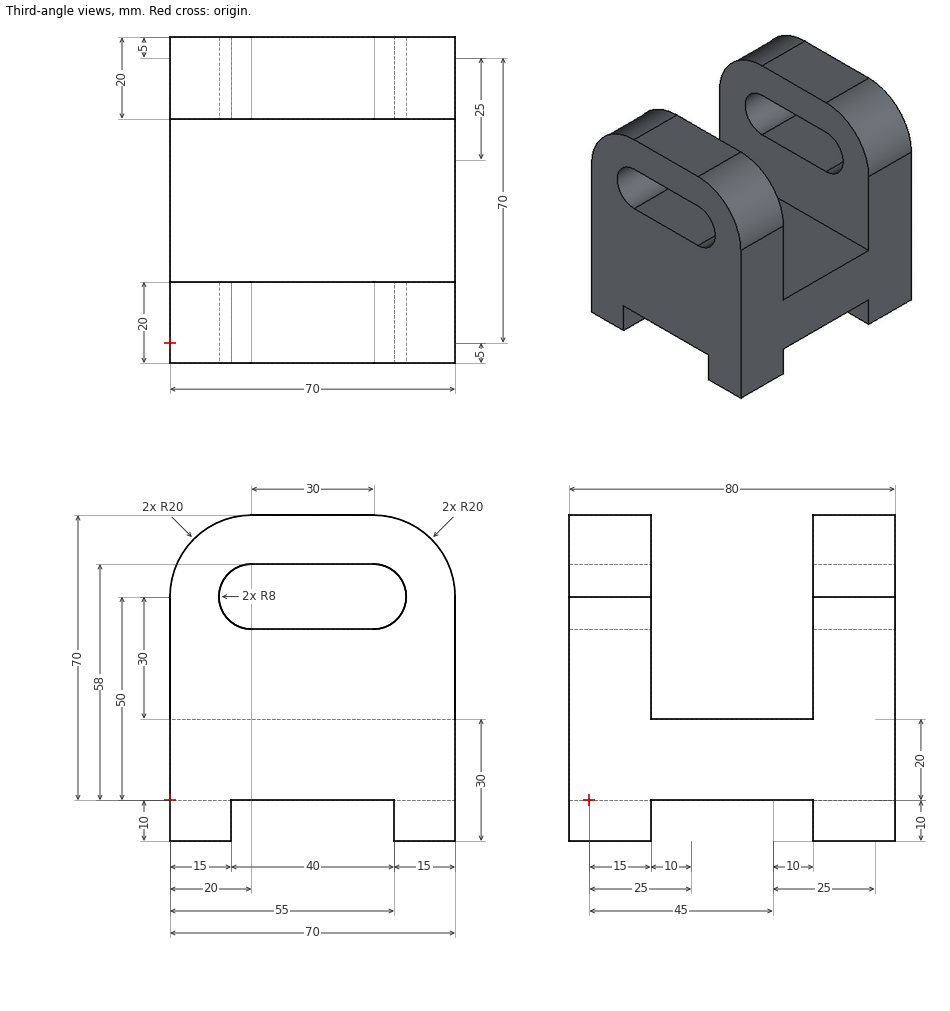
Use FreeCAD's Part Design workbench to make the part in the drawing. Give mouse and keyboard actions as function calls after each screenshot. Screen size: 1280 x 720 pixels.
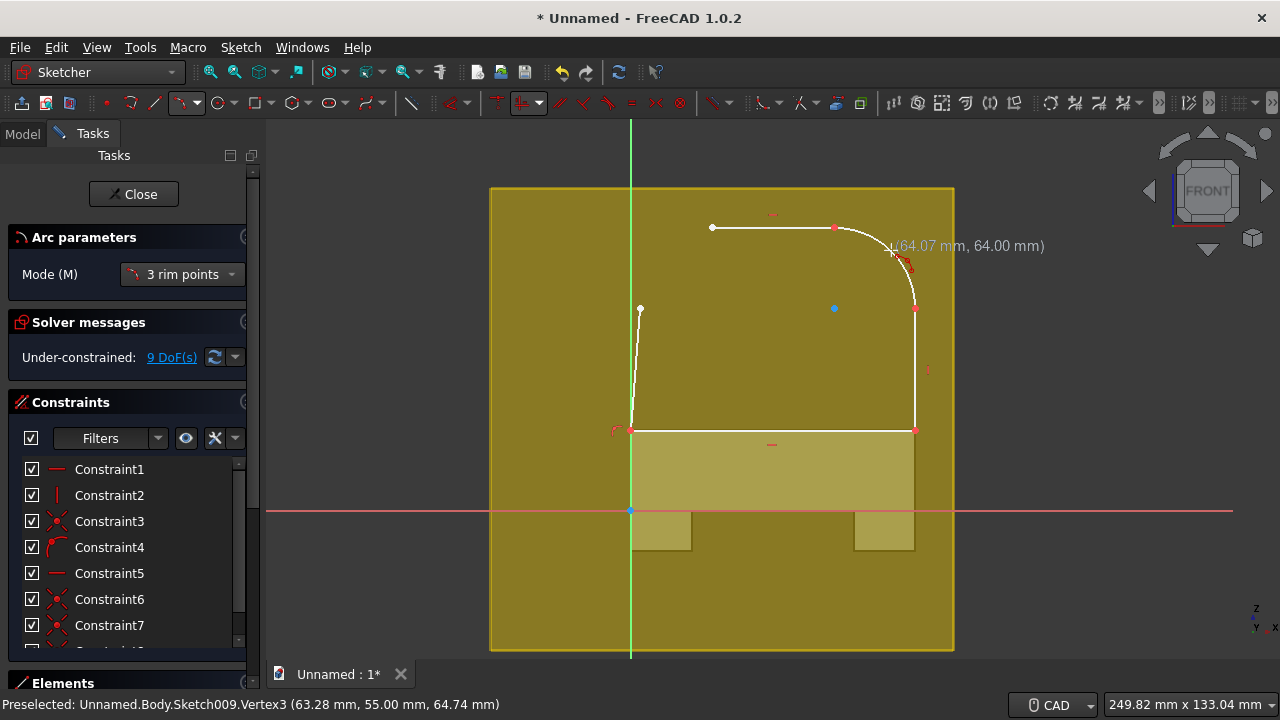
click(640, 309)
click(712, 228)
click(655, 250)
key(Escape)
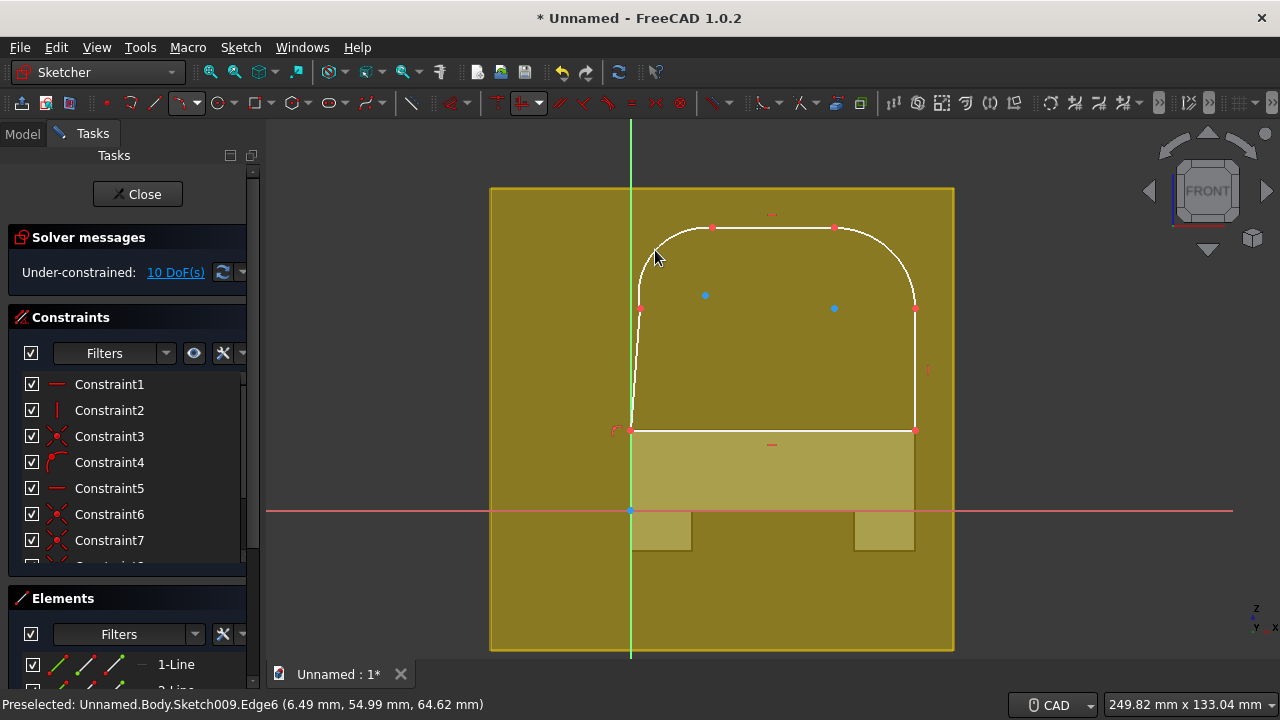
click(749, 228)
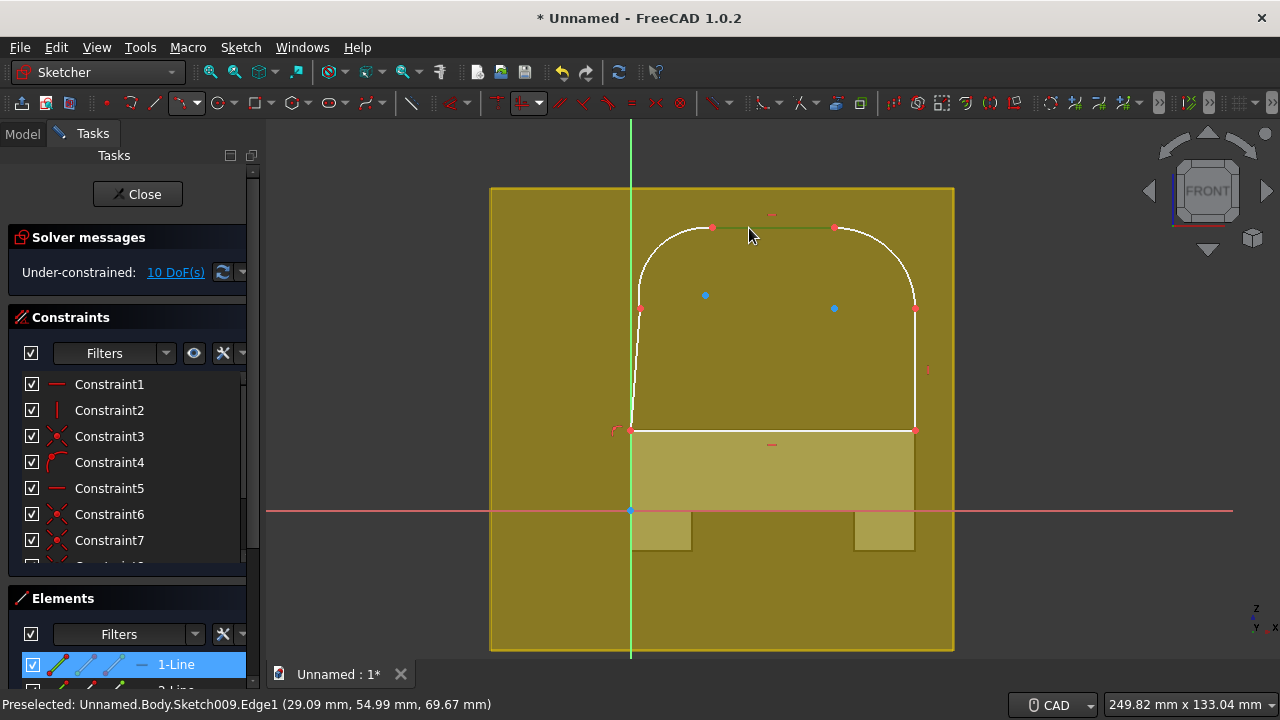
click(906, 272)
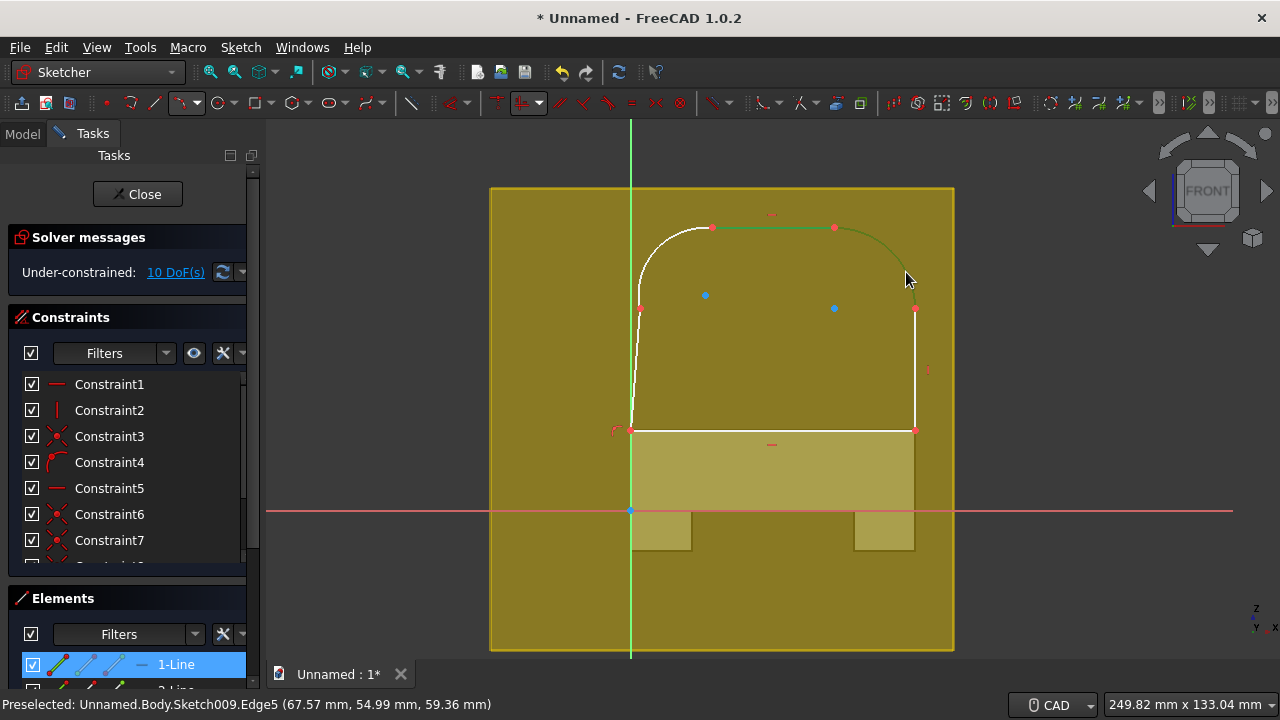
click(608, 104)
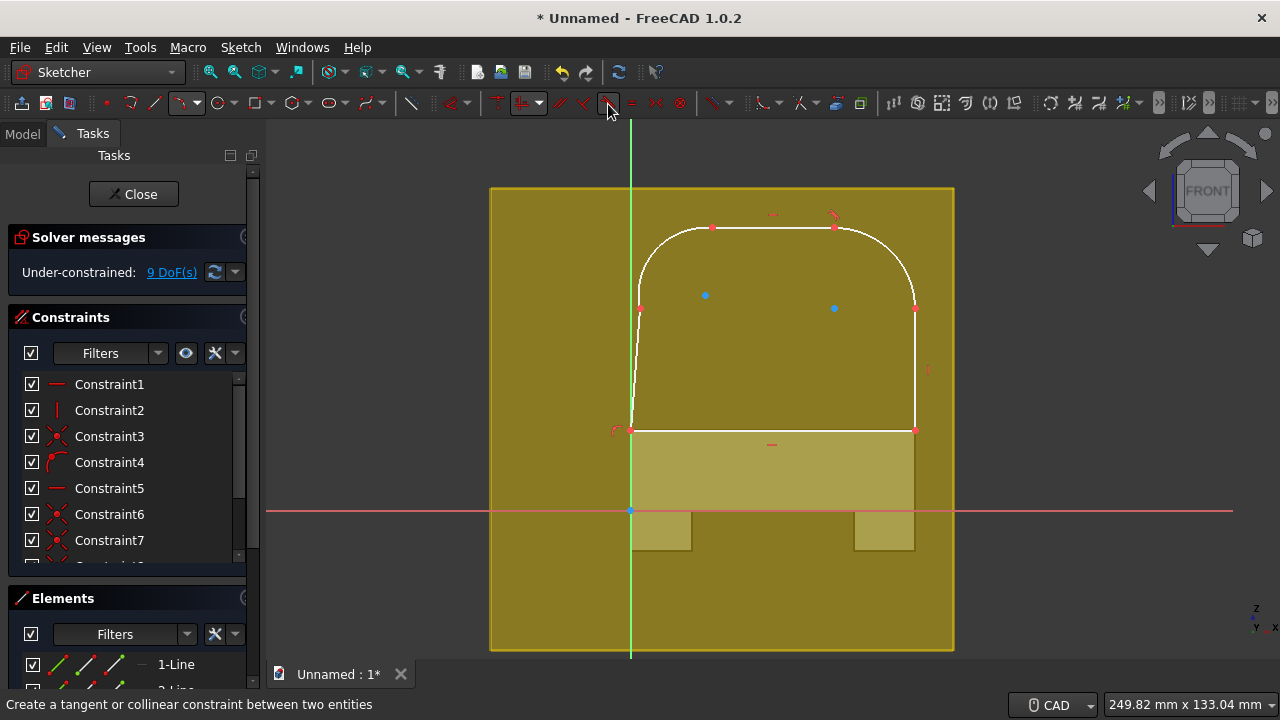
click(749, 228)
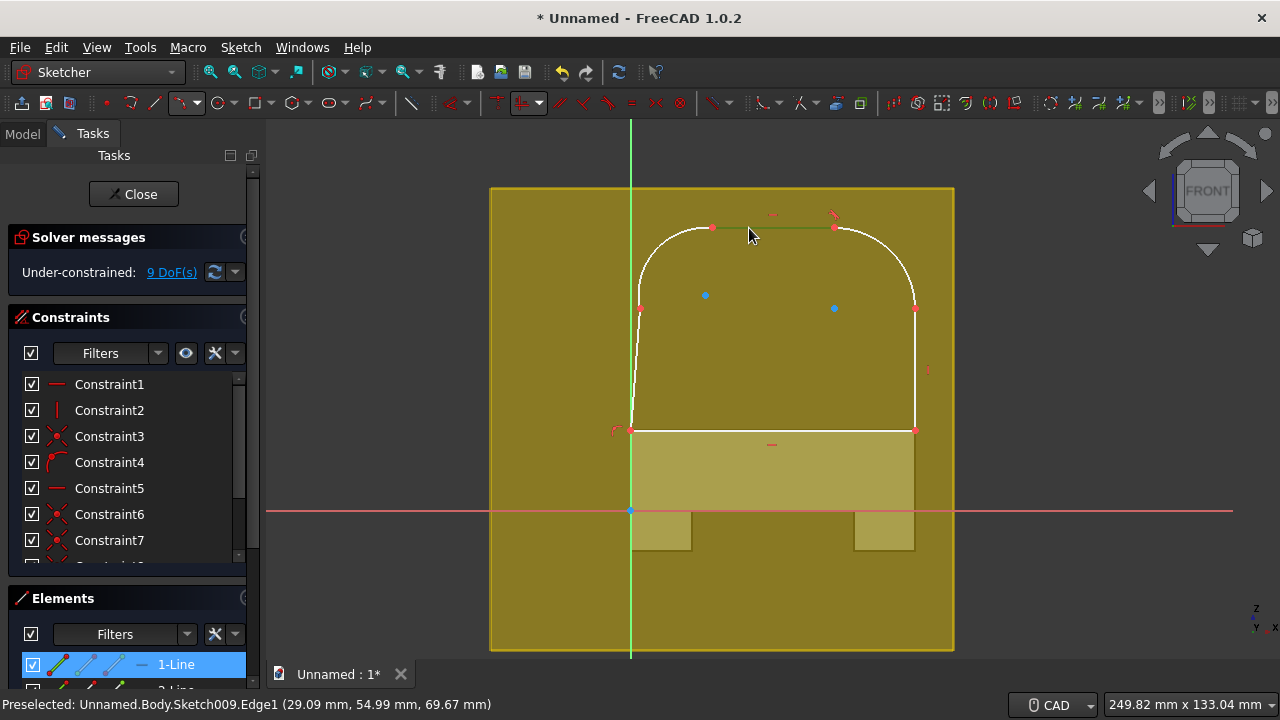
click(675, 235)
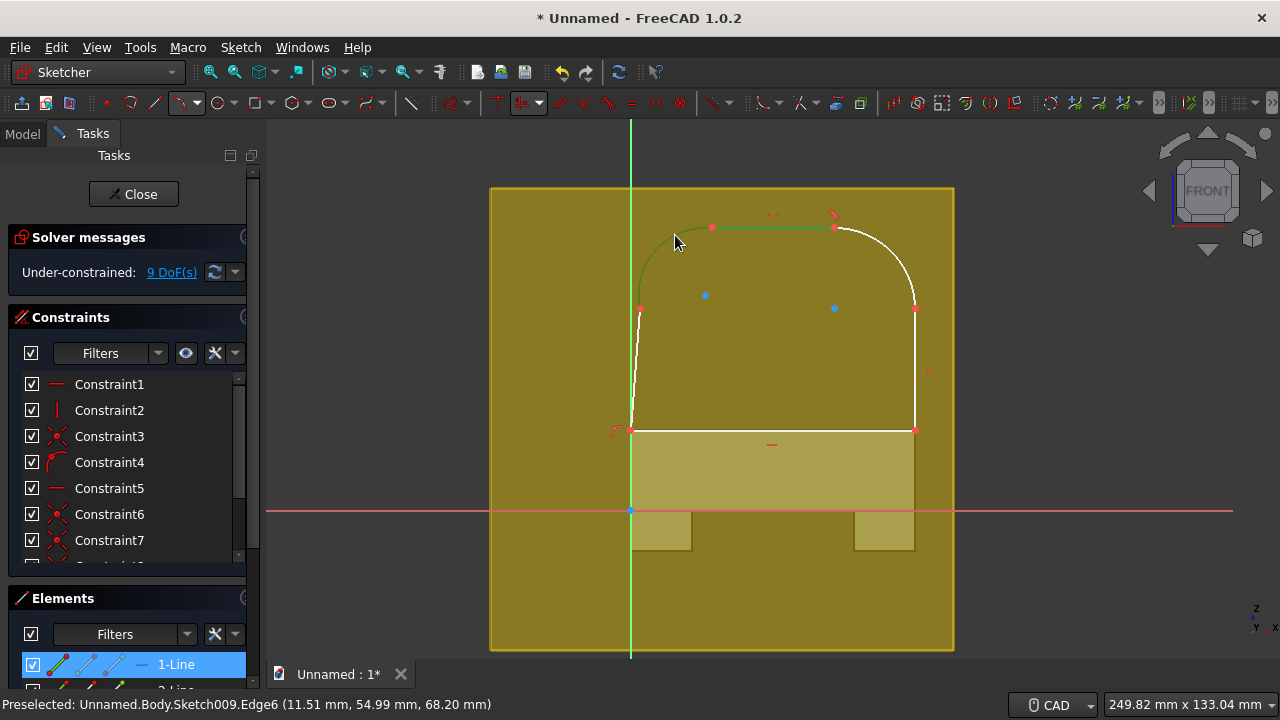
key(t)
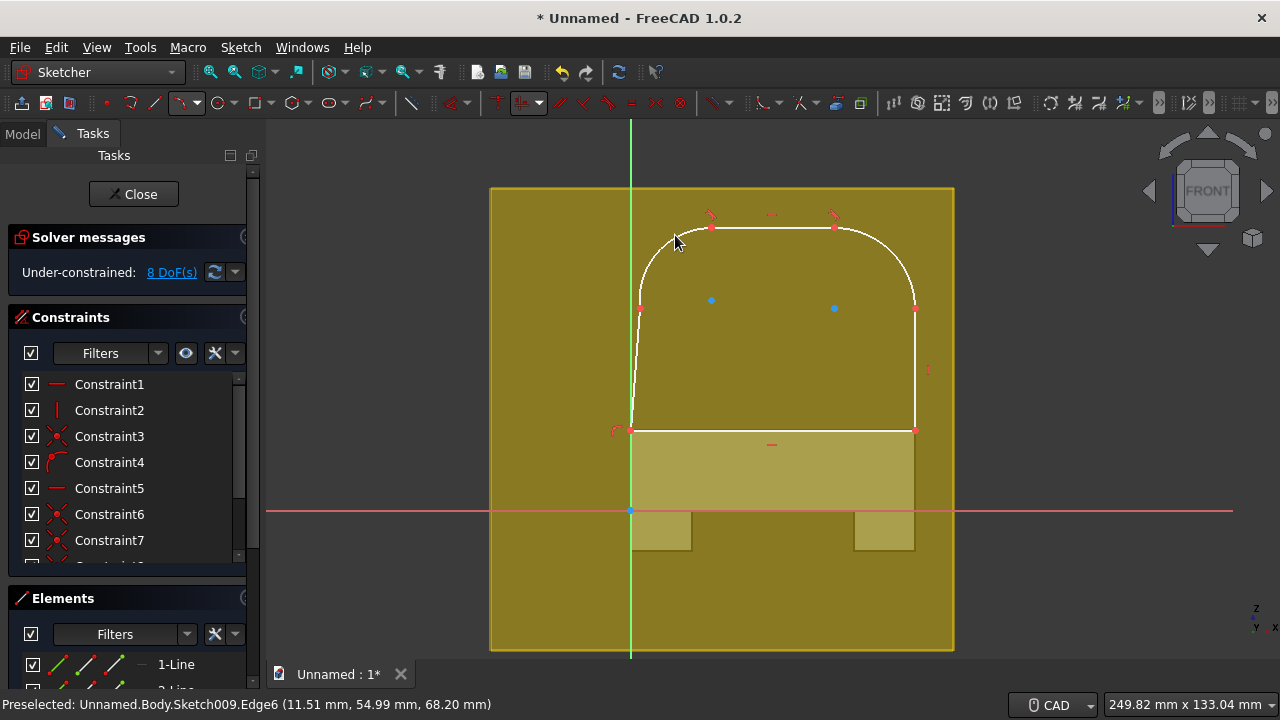
click(915, 346)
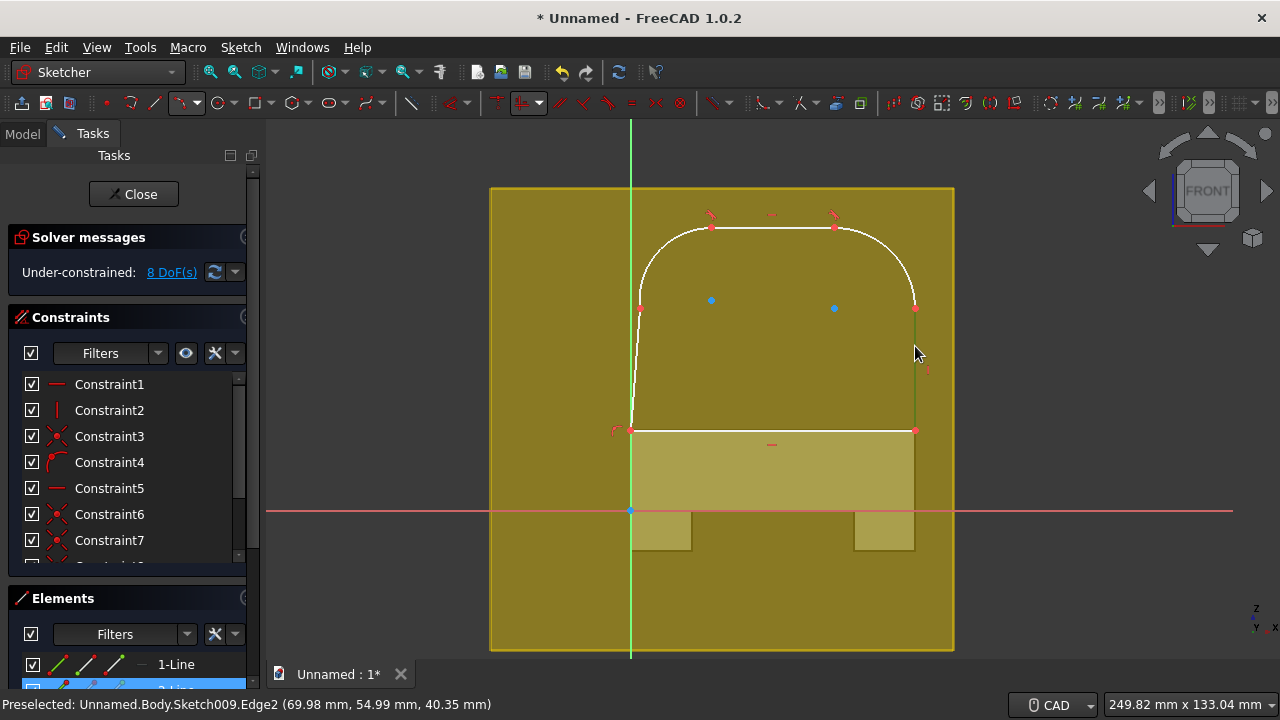
click(906, 272)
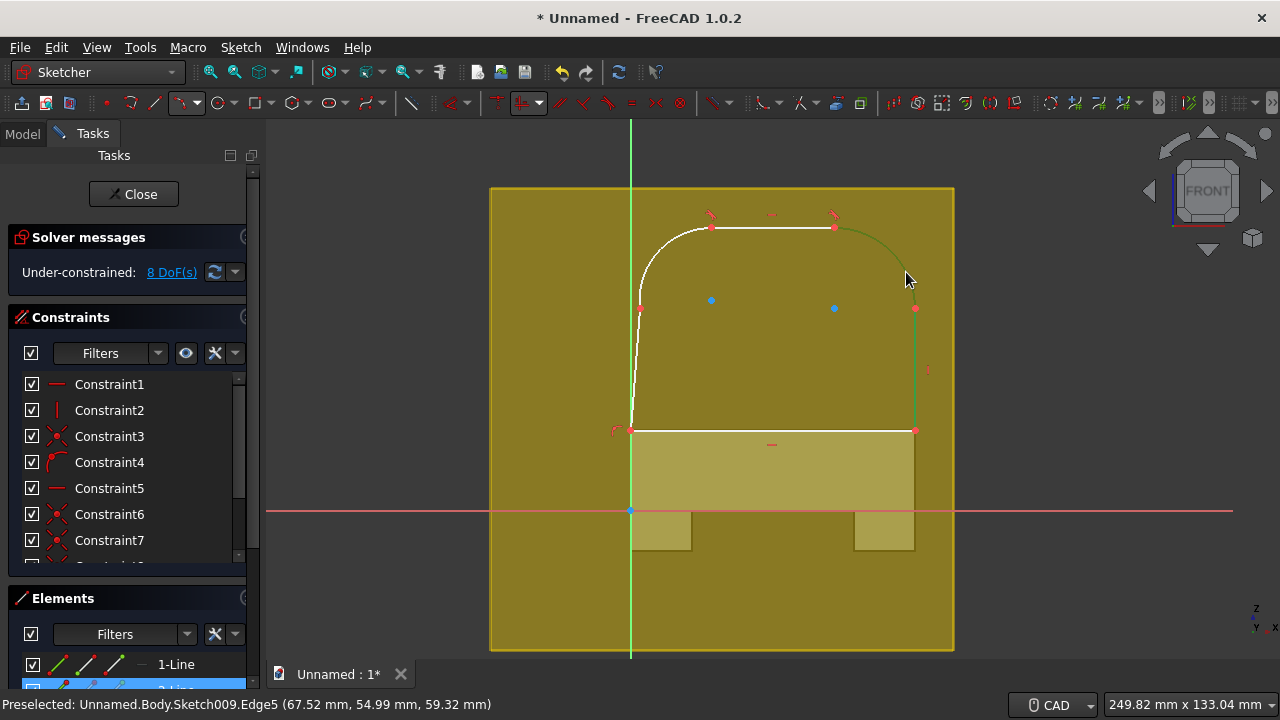
click(608, 104)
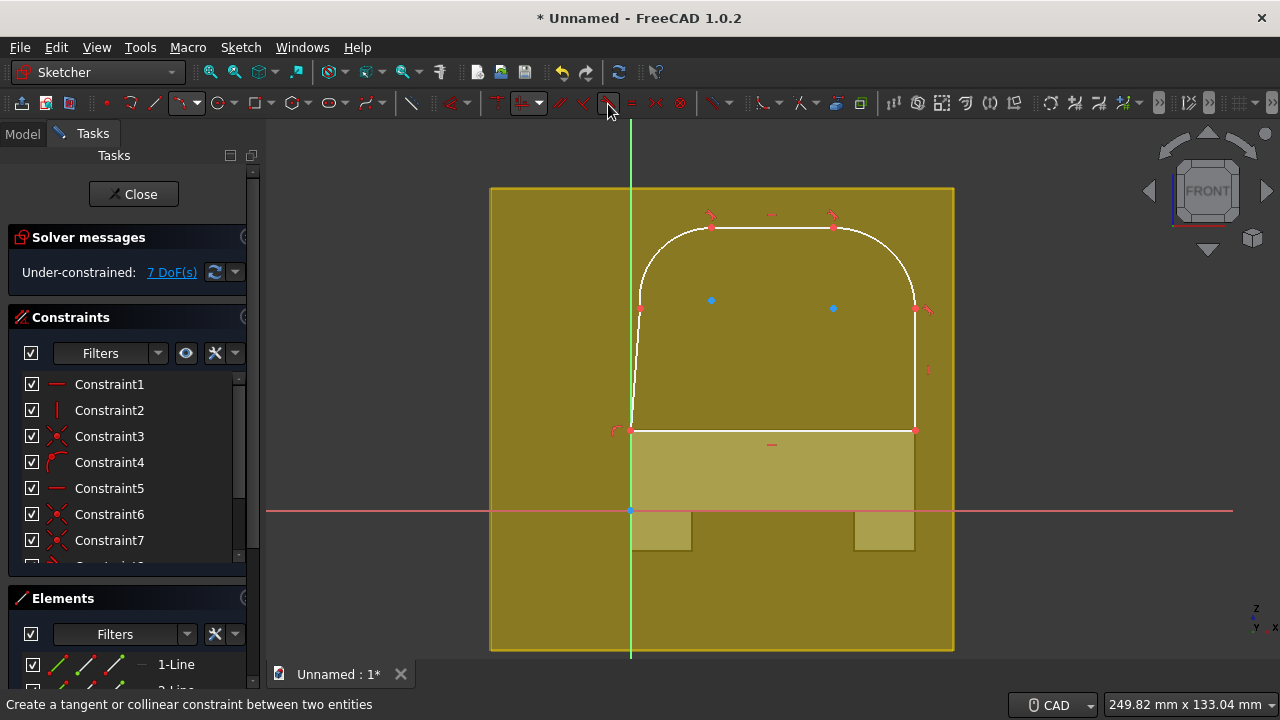
click(634, 394)